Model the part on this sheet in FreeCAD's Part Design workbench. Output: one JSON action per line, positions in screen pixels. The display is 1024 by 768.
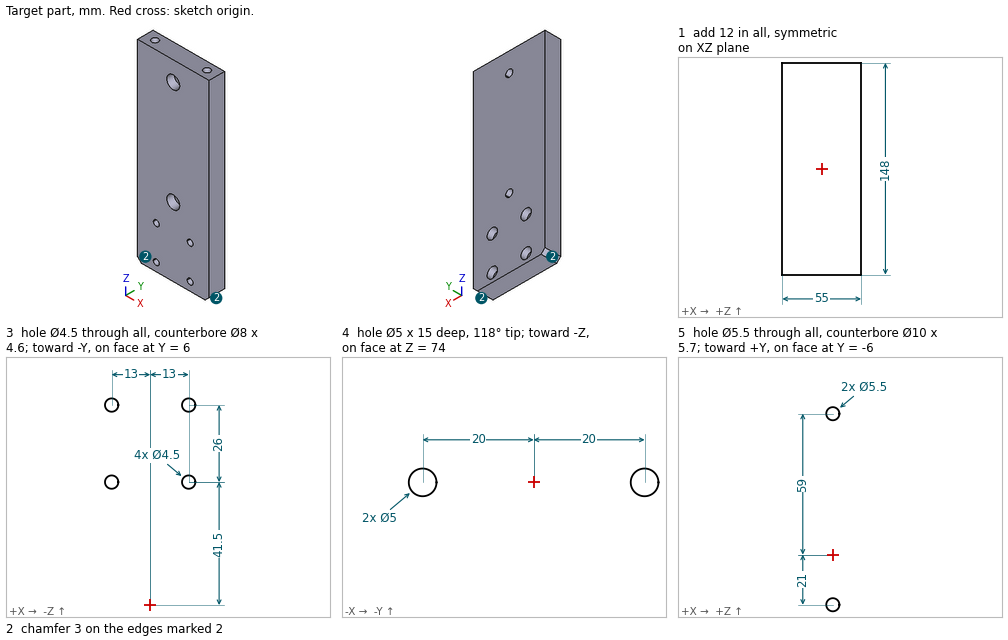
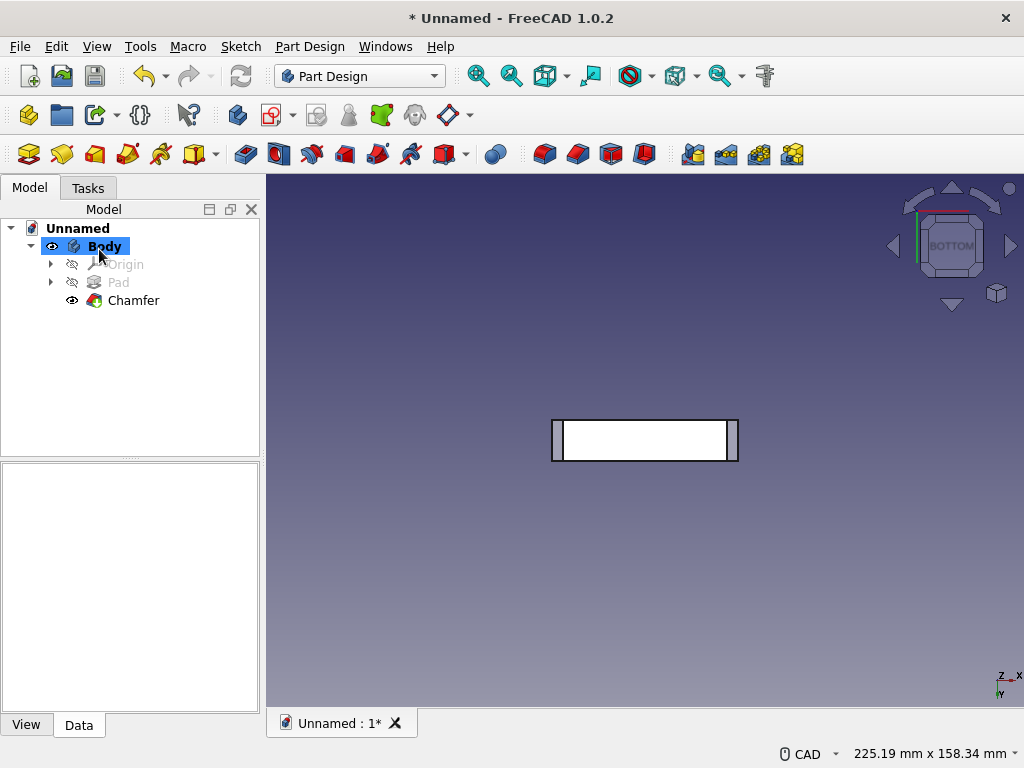
{"action": "key", "text": "v f"}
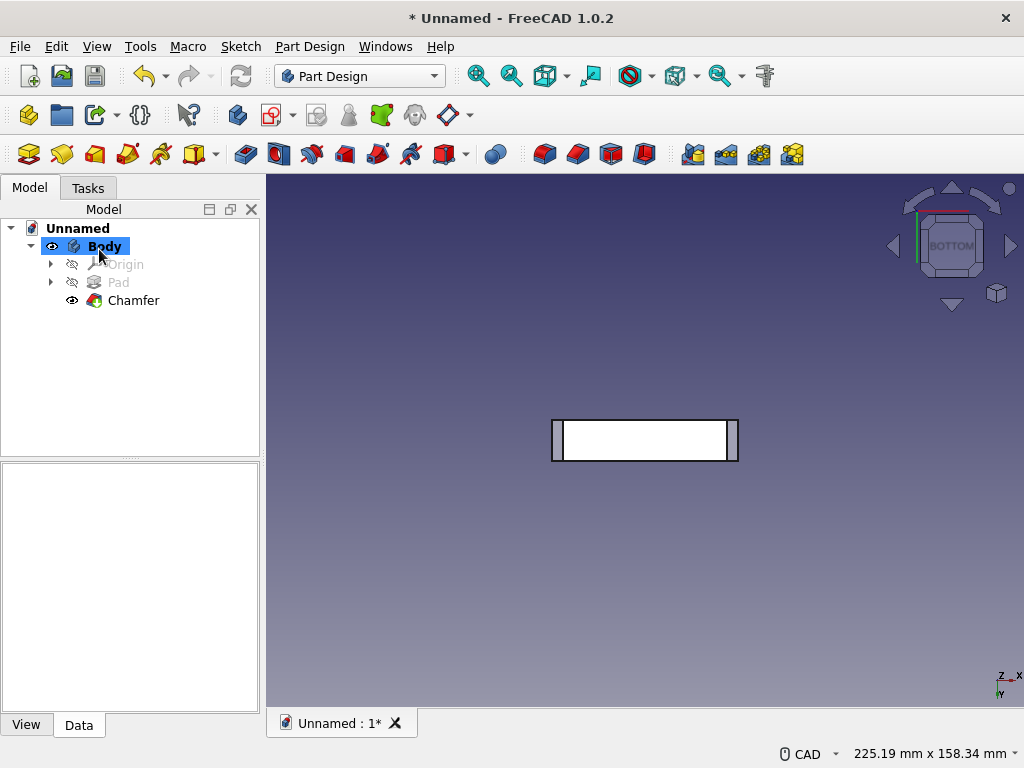
{"action": "key", "text": "4"}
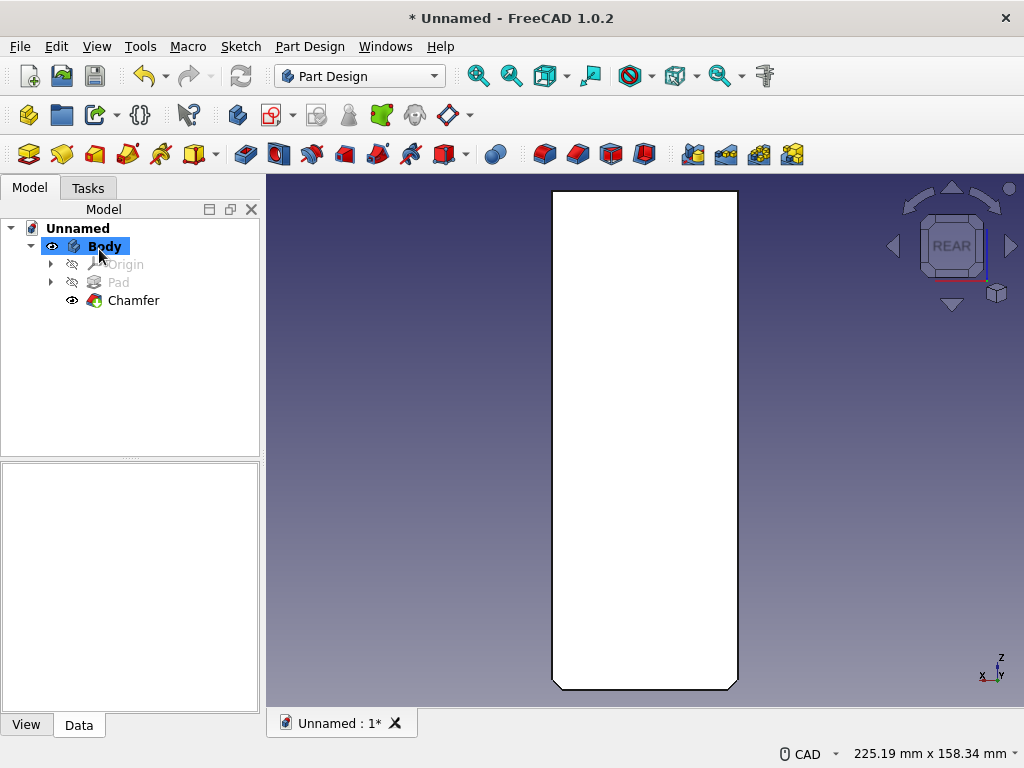
{"action": "left_click", "coordinate": [645, 297]}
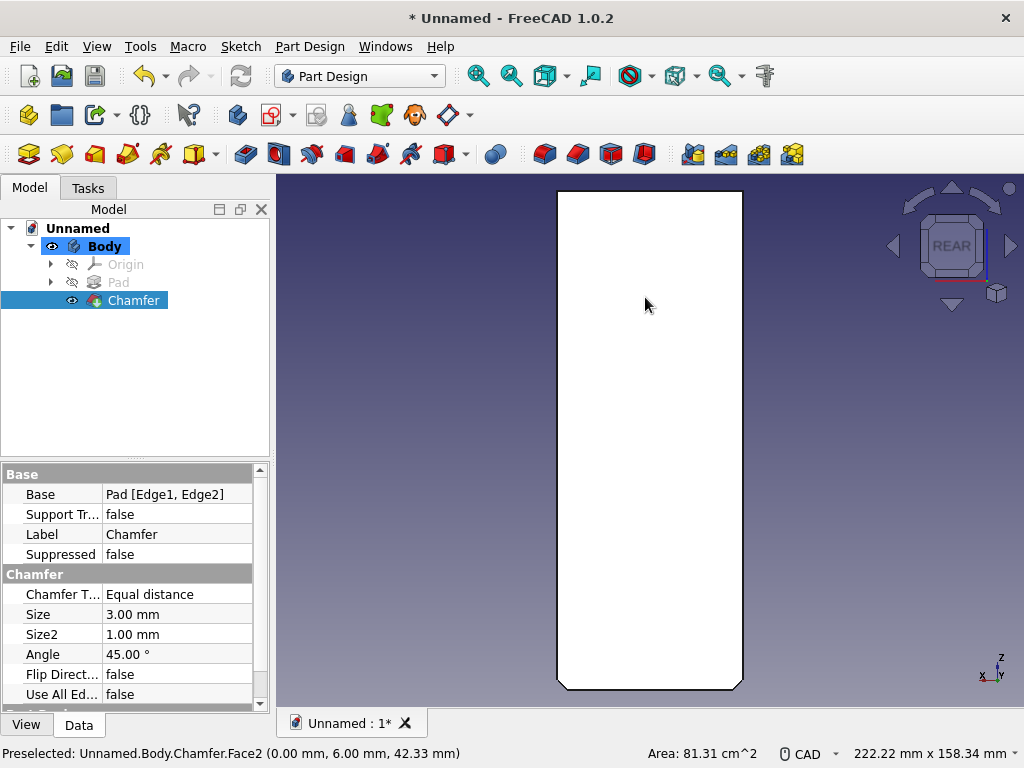
{"action": "left_click", "coordinate": [270, 116]}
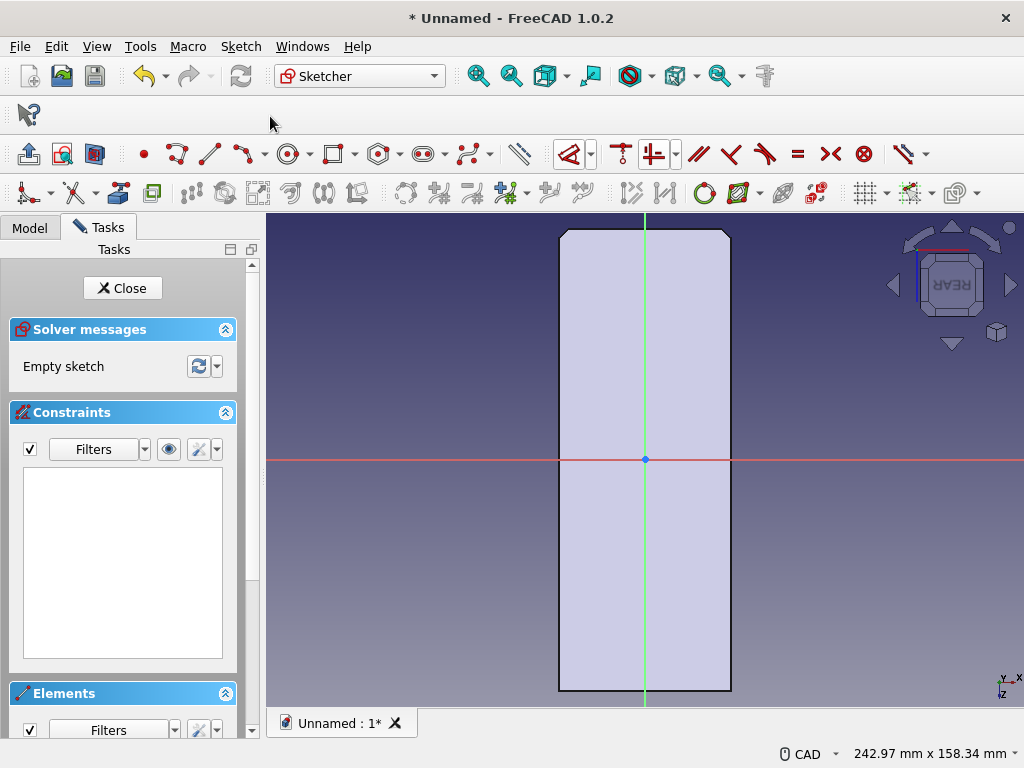
{"action": "scroll", "coordinate": [294, 679], "scroll_direction": "down", "scroll_amount": 1}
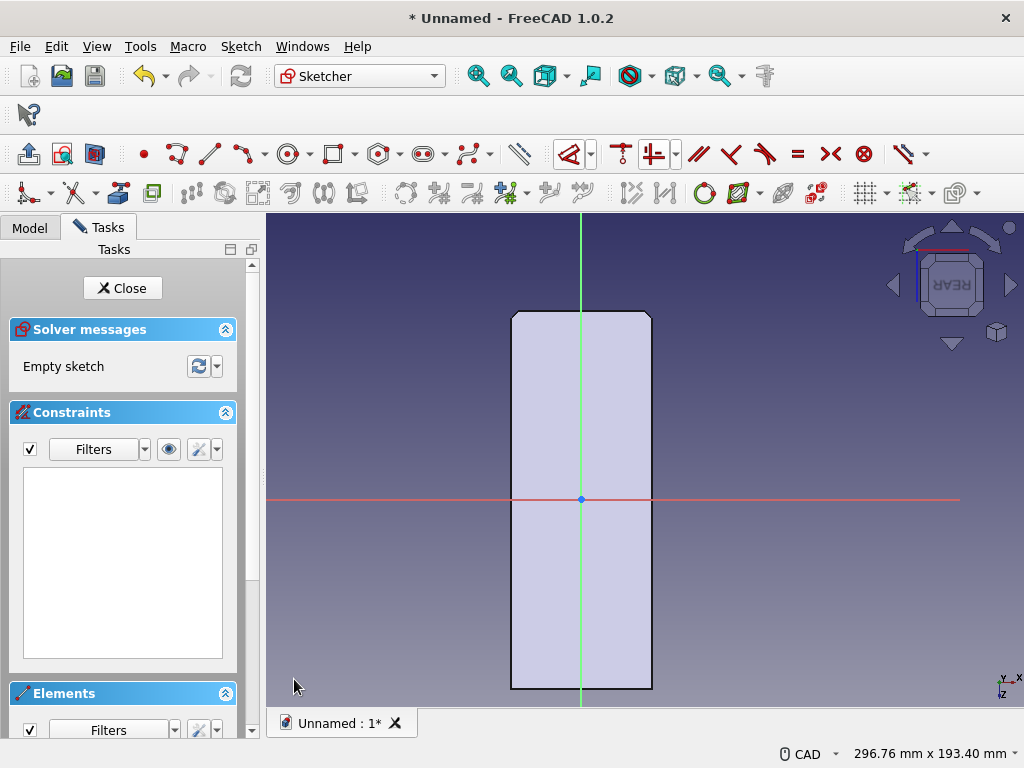
{"action": "scroll", "coordinate": [587, 351], "scroll_direction": "up", "scroll_amount": 3}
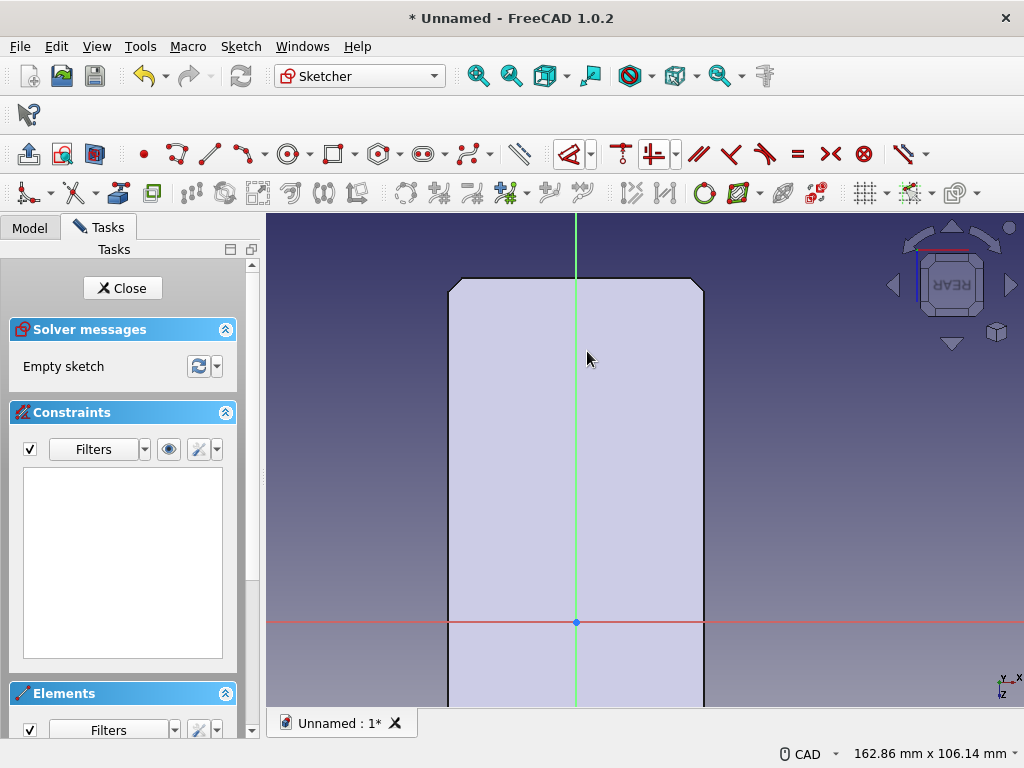
{"action": "key", "text": "g c"}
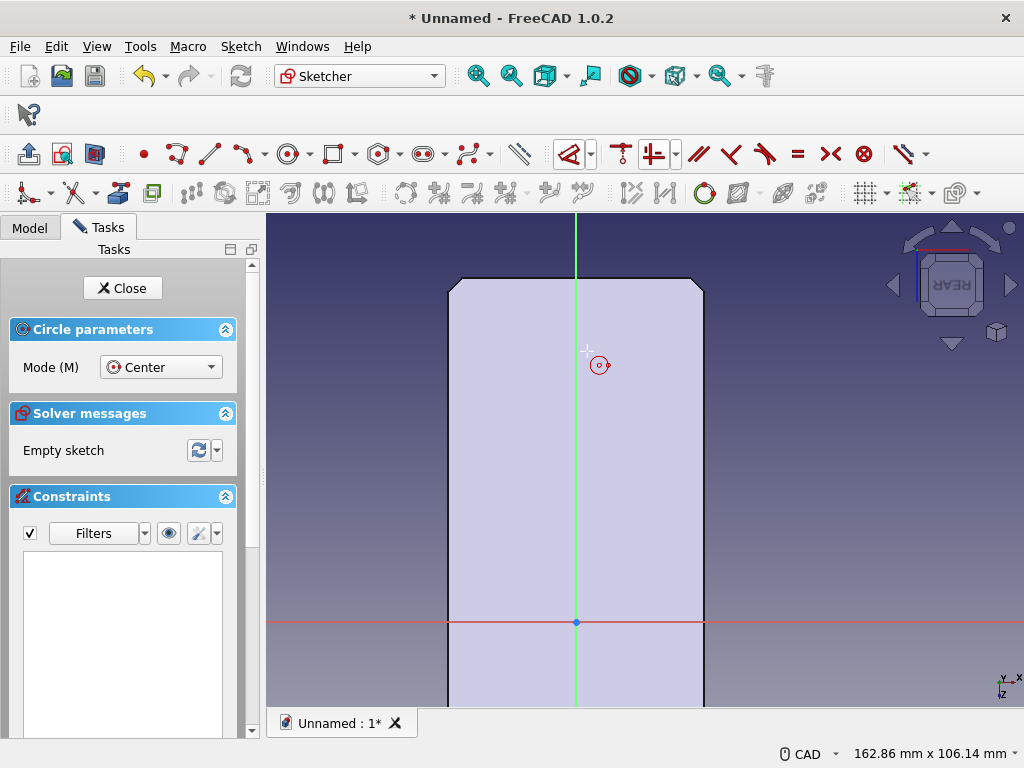
{"action": "scroll", "coordinate": [637, 429], "scroll_direction": "up", "scroll_amount": 4}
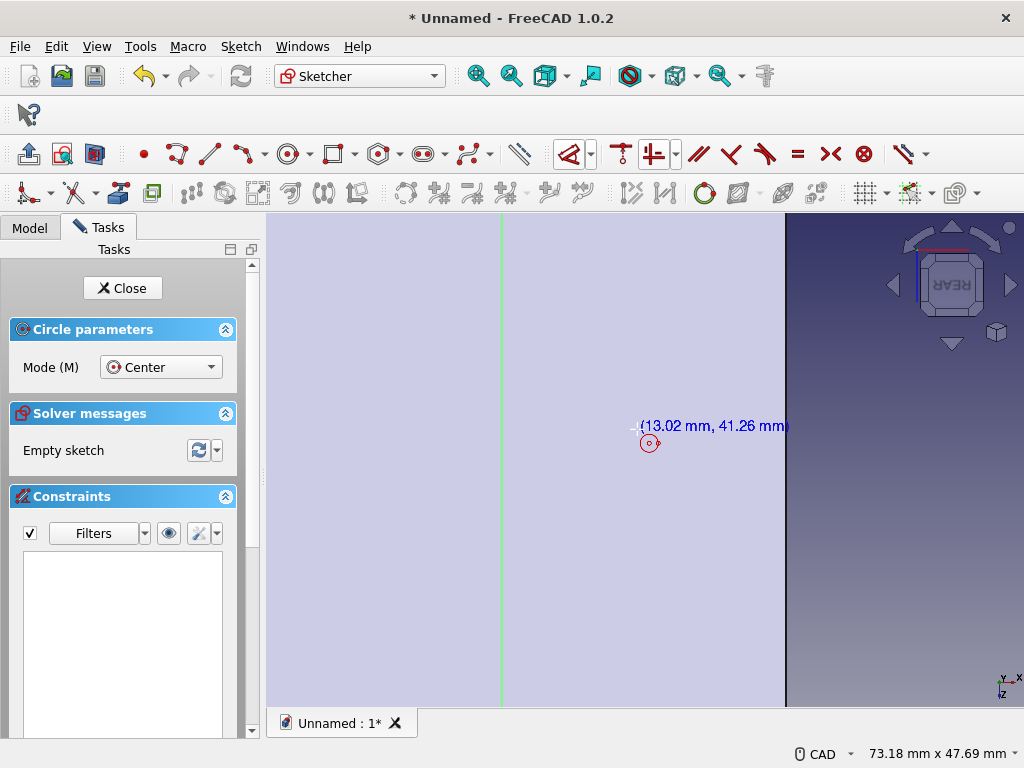
{"action": "left_click", "coordinate": [636, 428]}
{"action": "mouse_move", "coordinate": [653, 412]}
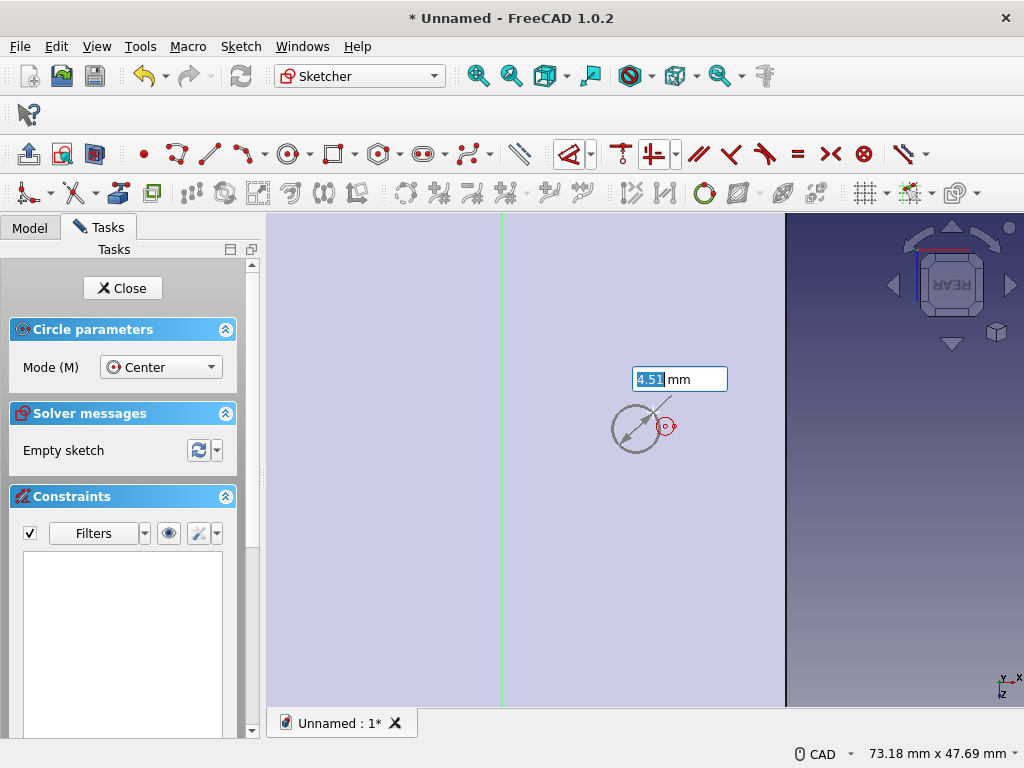
{"action": "type", "text": "4.5"}
{"action": "key", "text": "Return"}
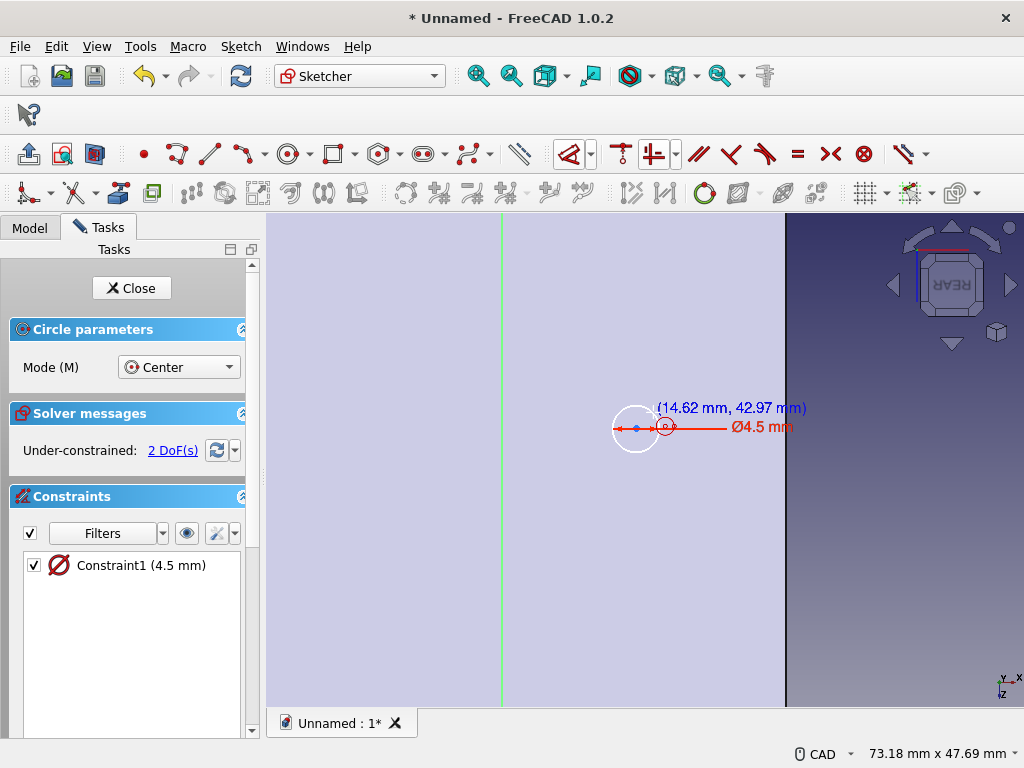
{"action": "scroll", "coordinate": [638, 430], "scroll_direction": "down", "scroll_amount": 4}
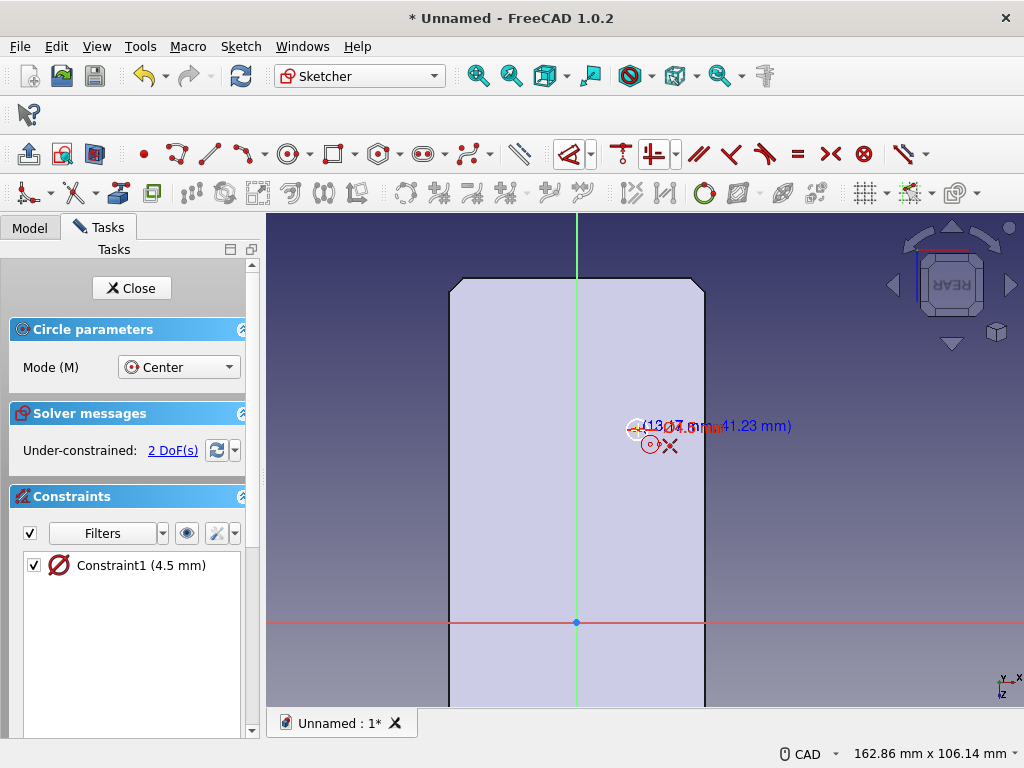
{"action": "scroll", "coordinate": [637, 308], "scroll_direction": "up", "scroll_amount": 4}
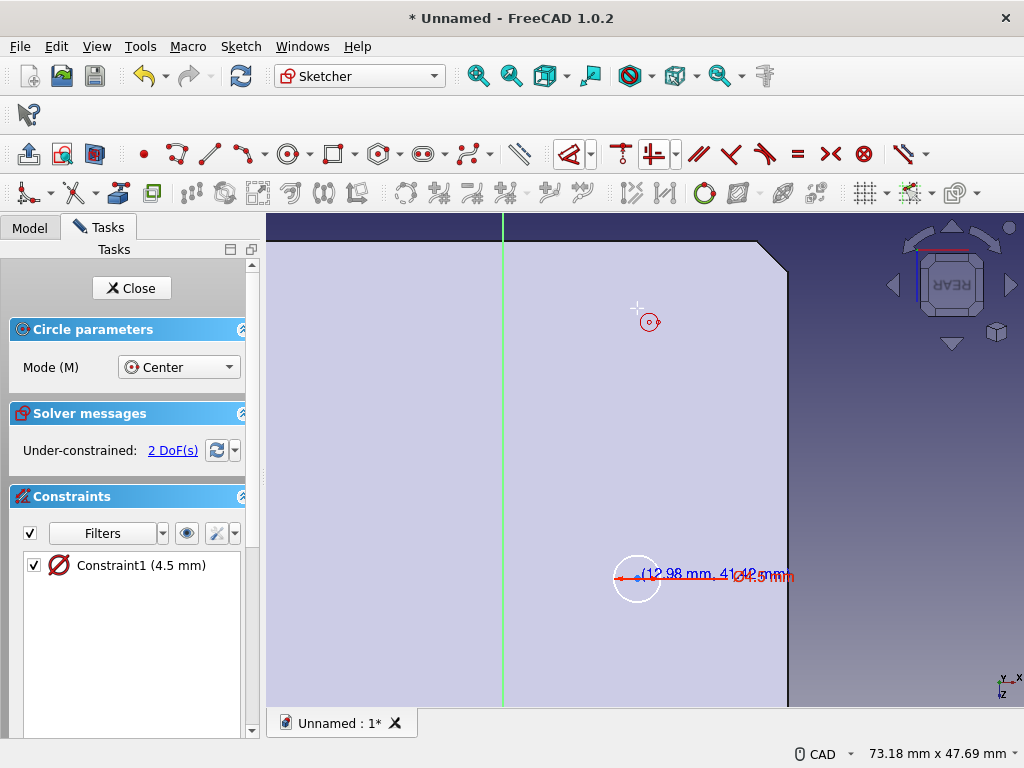
{"action": "left_click", "coordinate": [637, 309]}
{"action": "mouse_move", "coordinate": [654, 292]}